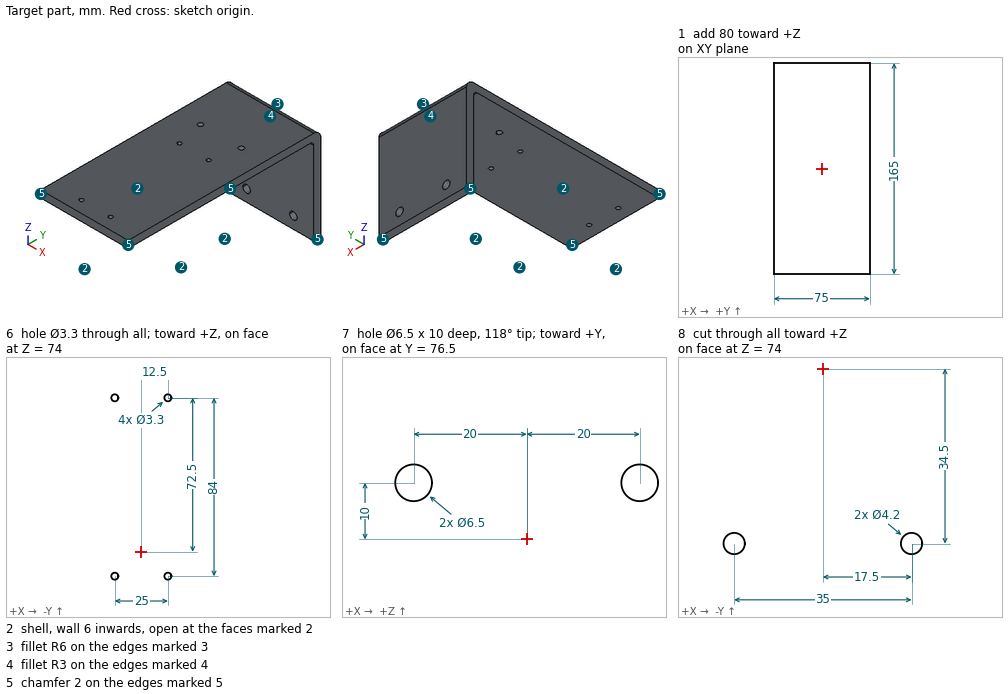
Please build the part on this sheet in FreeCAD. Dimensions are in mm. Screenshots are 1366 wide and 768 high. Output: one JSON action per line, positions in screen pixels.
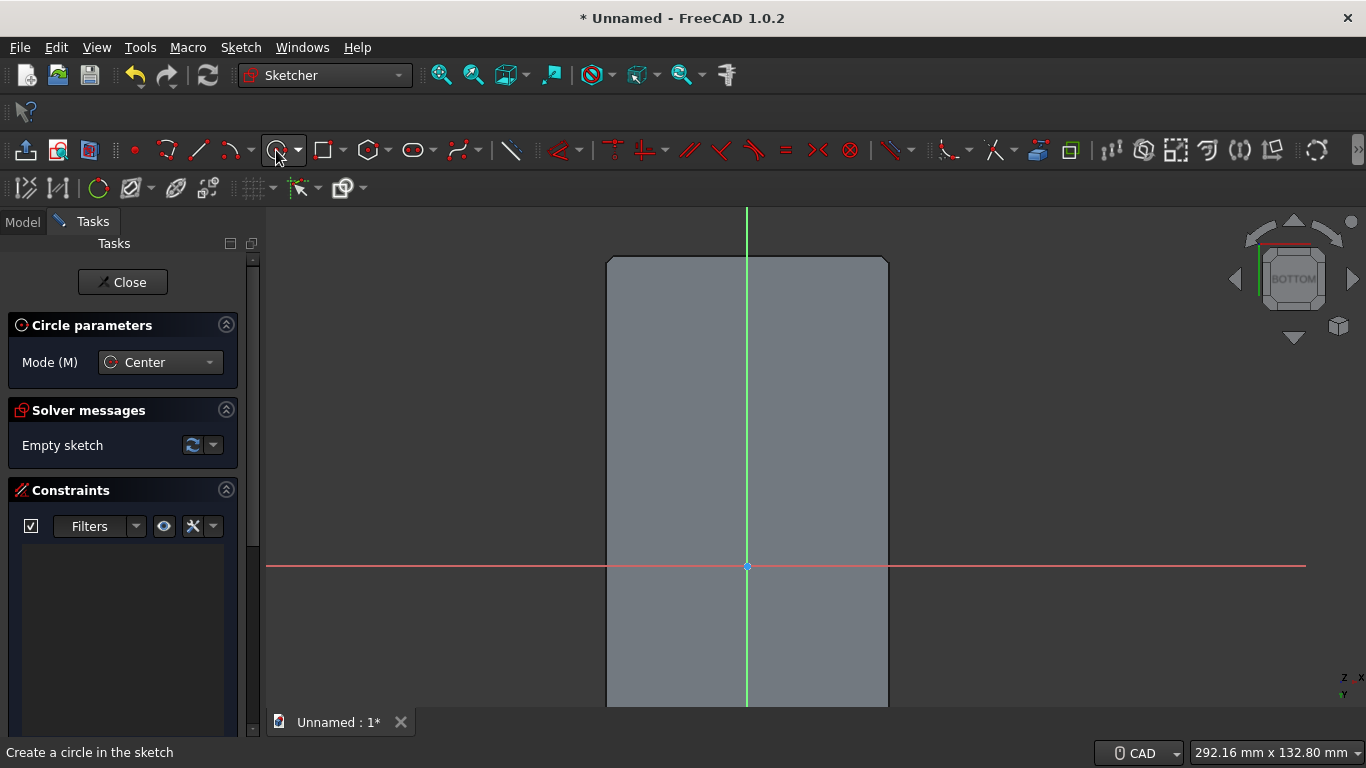
{"action": "scroll", "coordinate": [794, 293], "scroll_direction": "up", "scroll_amount": 7}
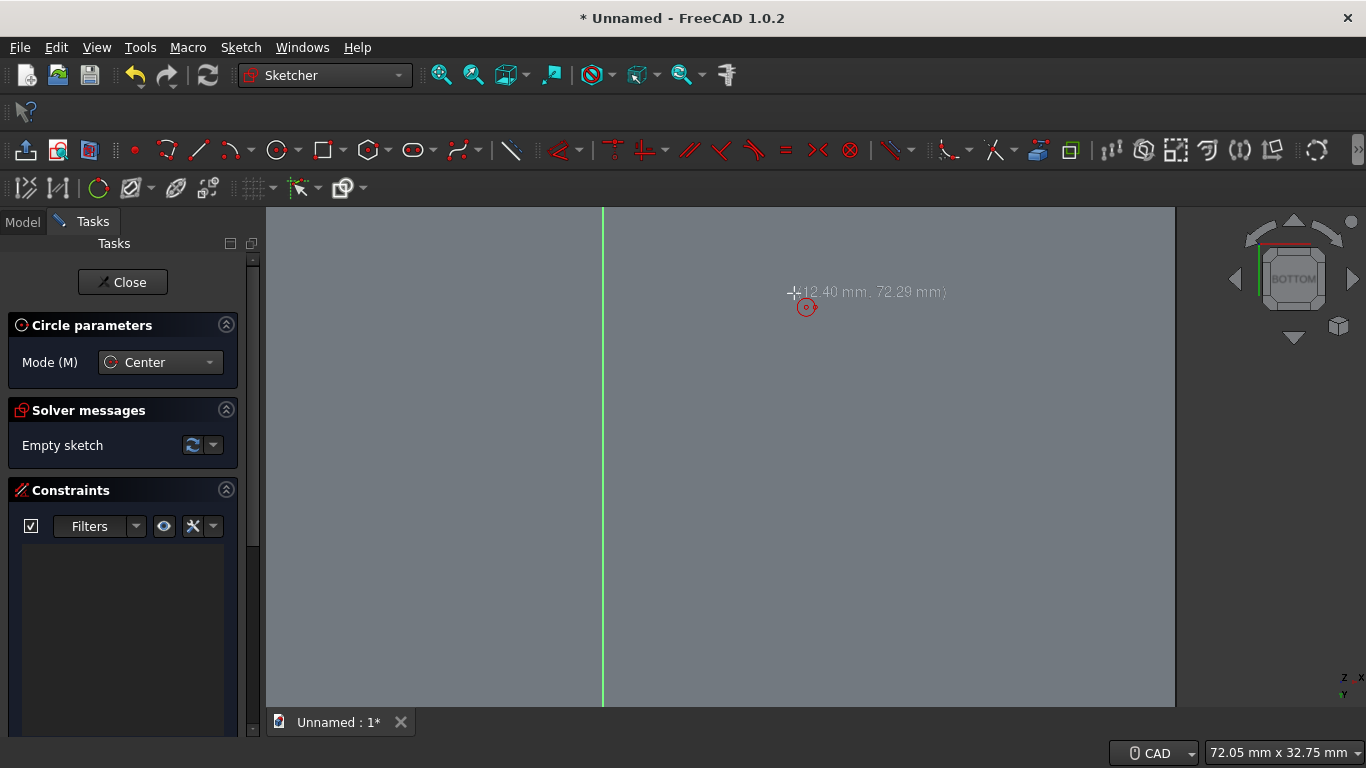
{"action": "scroll", "coordinate": [795, 301], "scroll_direction": "down", "scroll_amount": 7}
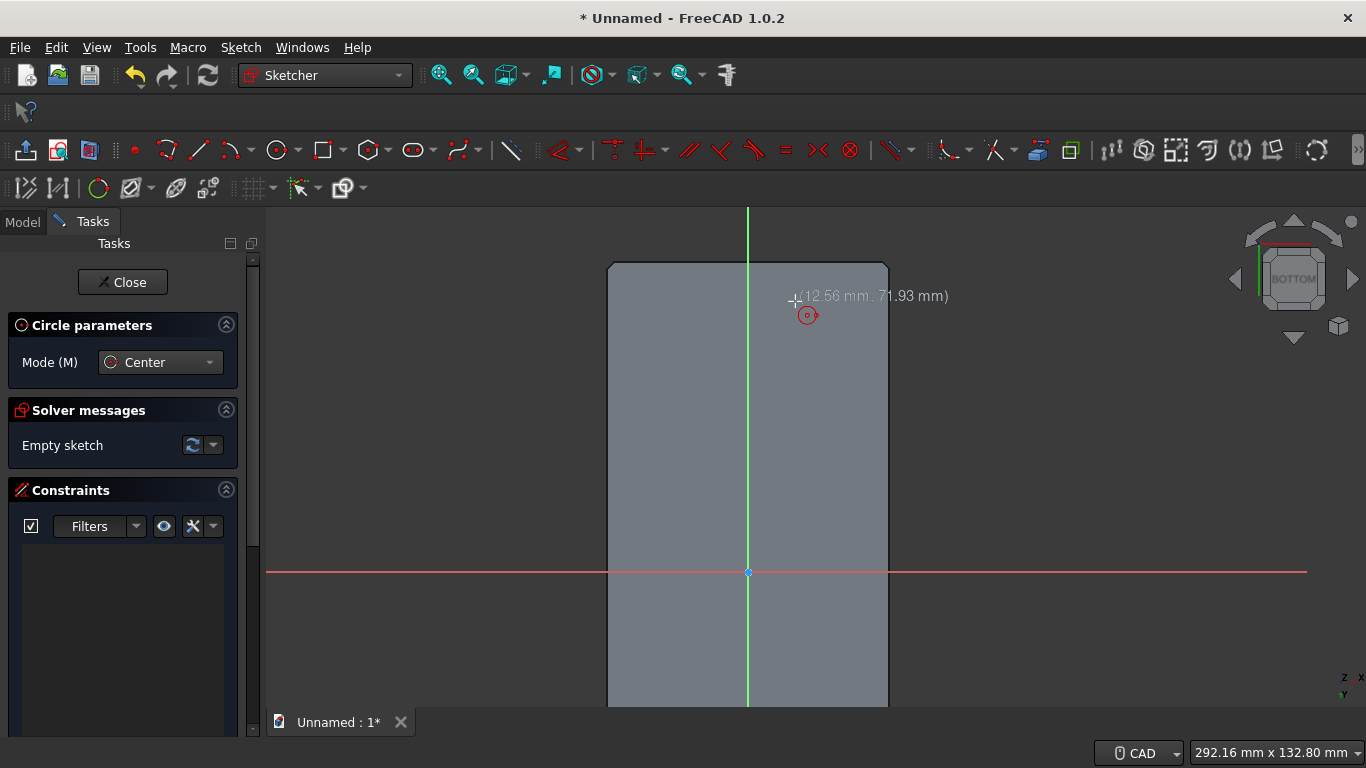
{"action": "left_click", "coordinate": [795, 299]}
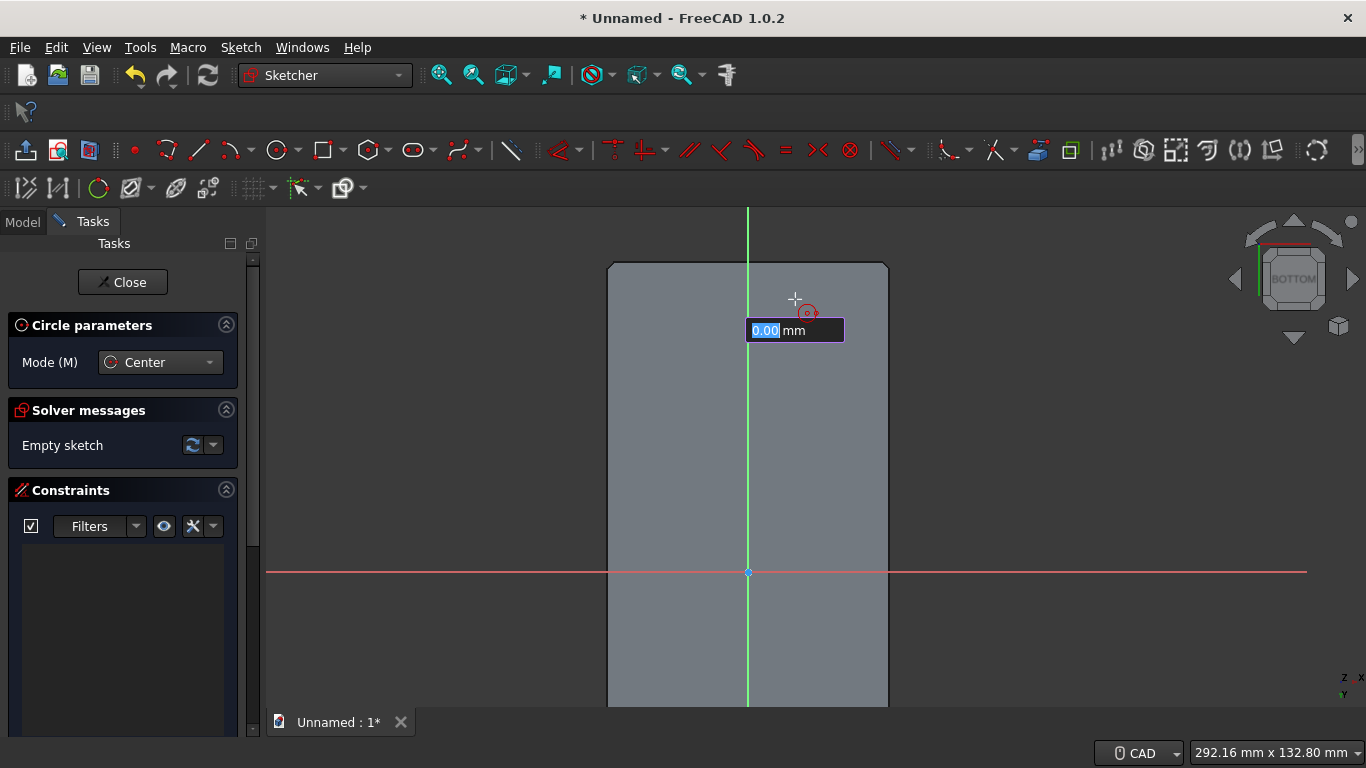
{"action": "scroll", "coordinate": [800, 295], "scroll_direction": "up", "scroll_amount": 5}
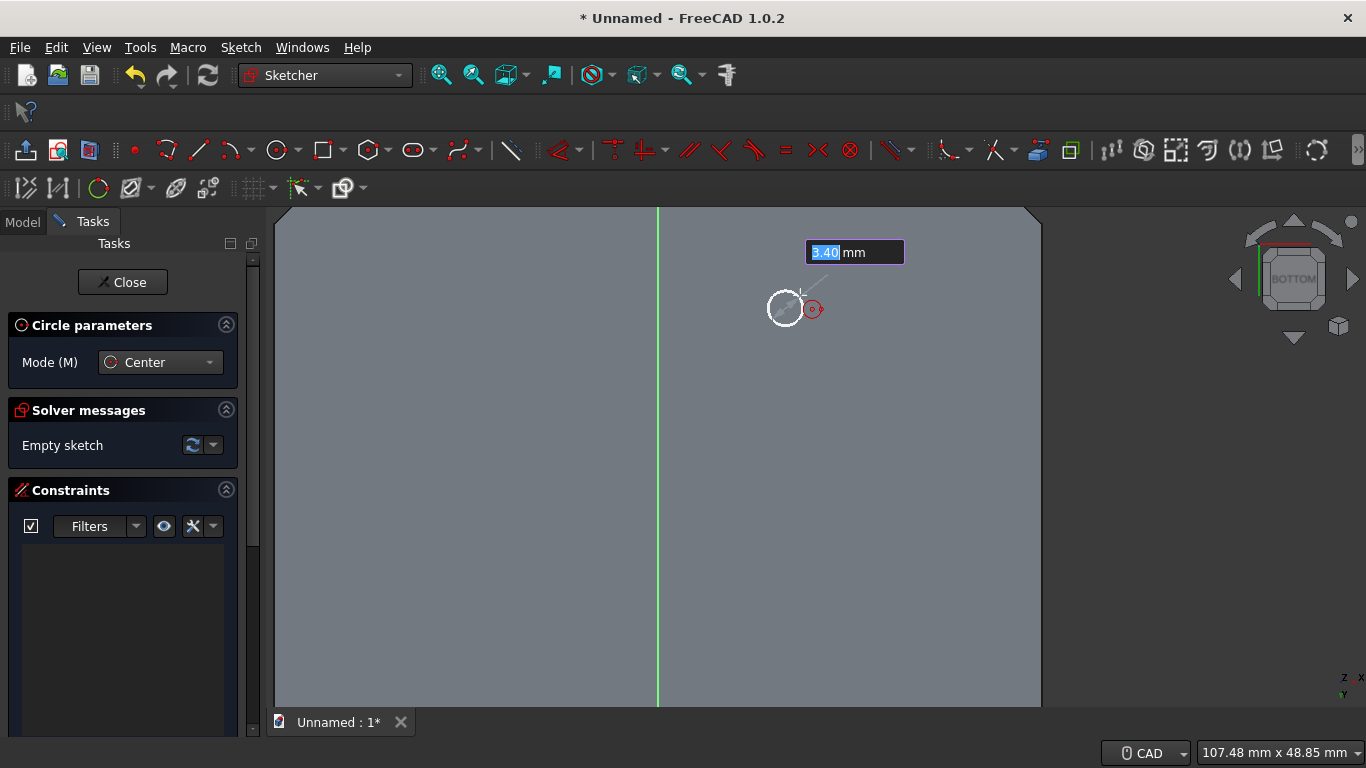
{"action": "left_click", "coordinate": [798, 294]}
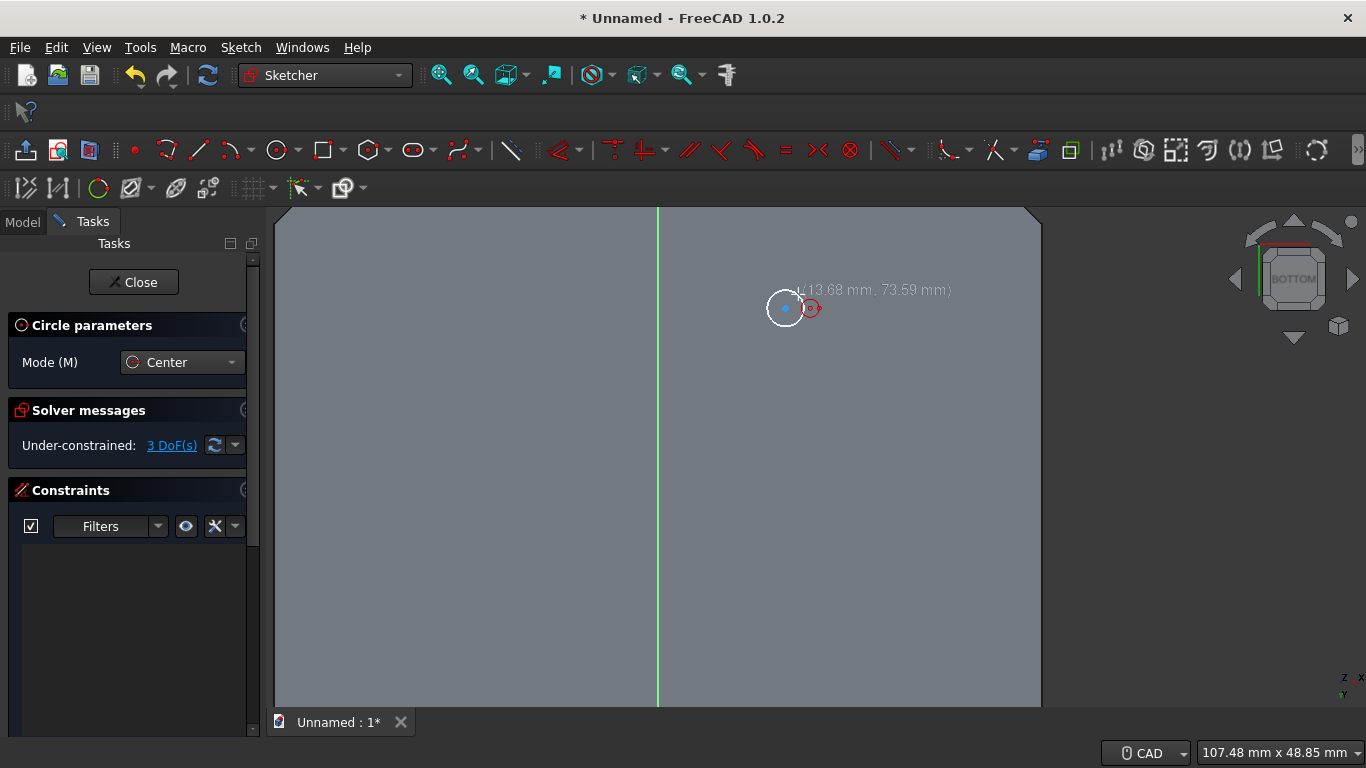
{"action": "scroll", "coordinate": [800, 295], "scroll_direction": "down", "scroll_amount": 5}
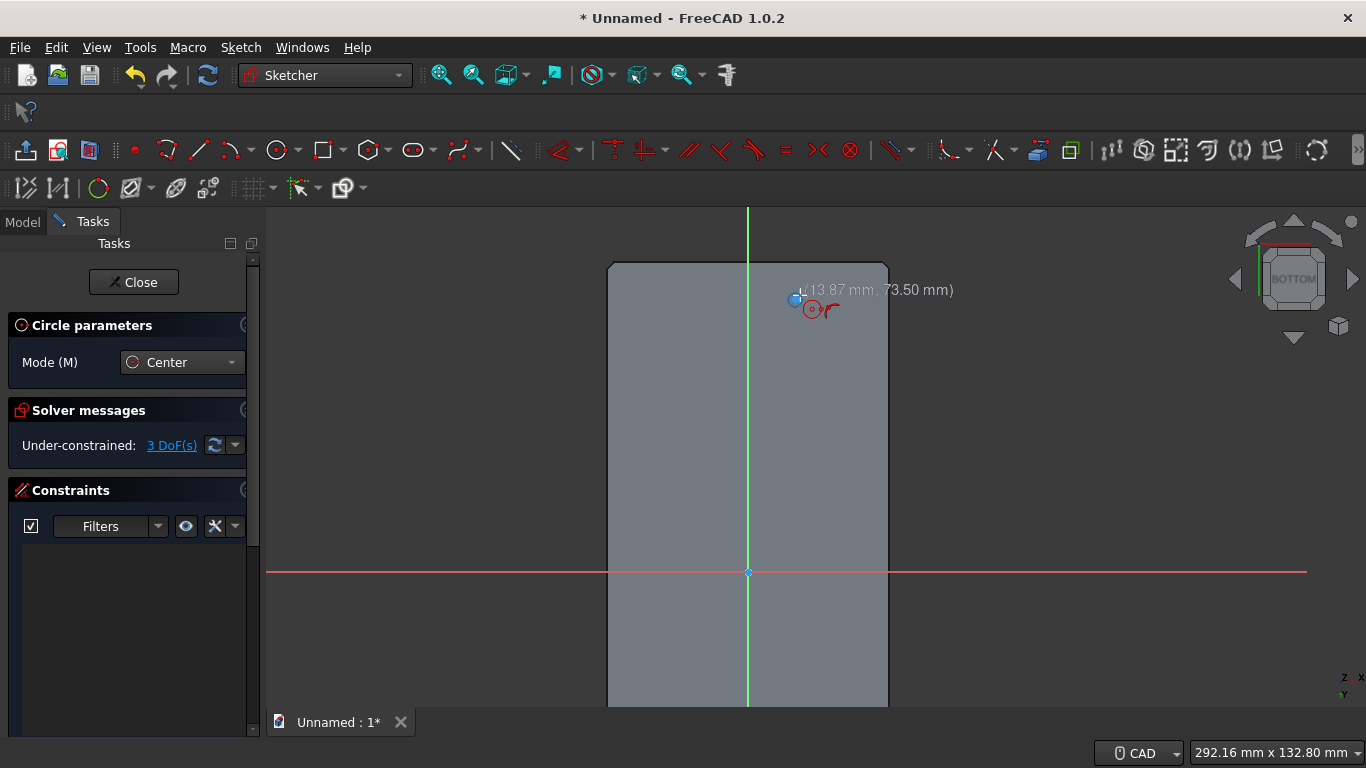
{"action": "scroll", "coordinate": [795, 615], "scroll_direction": "up", "scroll_amount": 7}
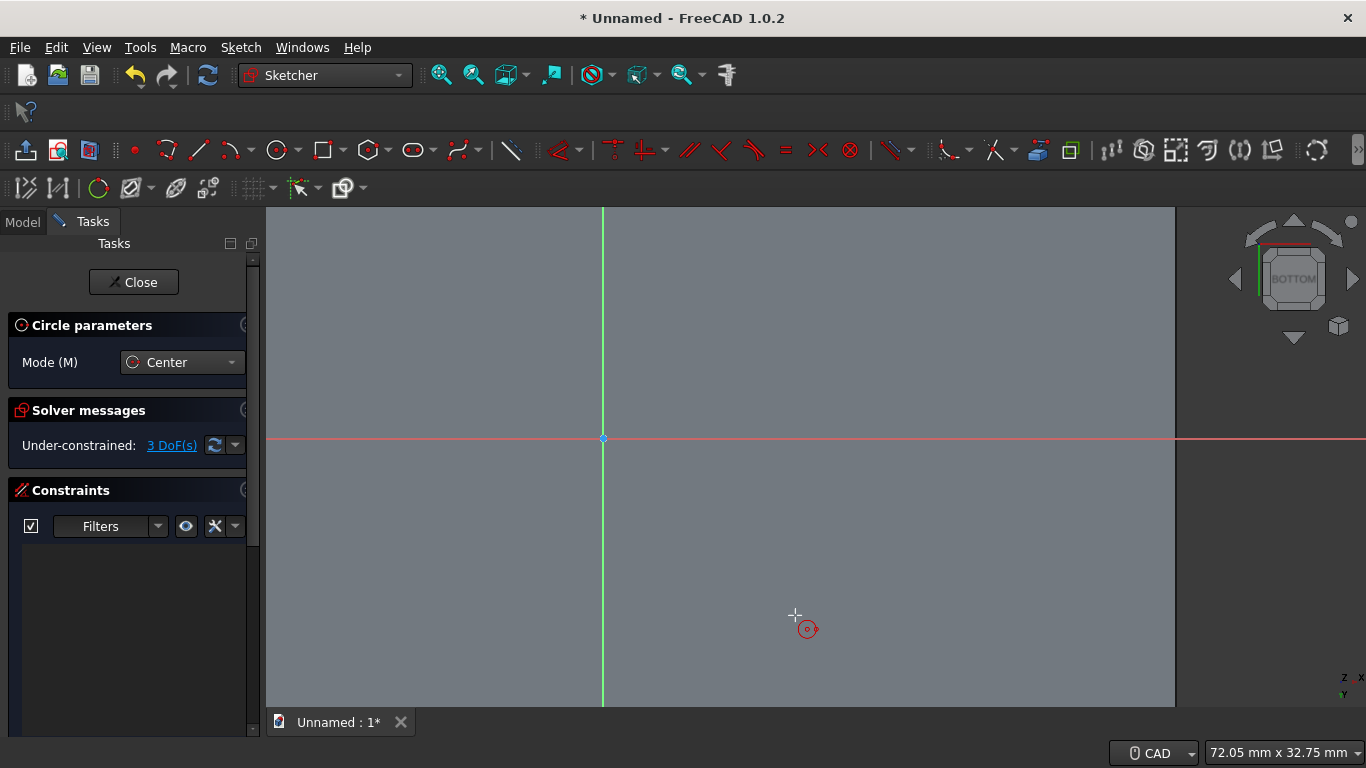
{"action": "scroll", "coordinate": [795, 615], "scroll_direction": "down", "scroll_amount": 7}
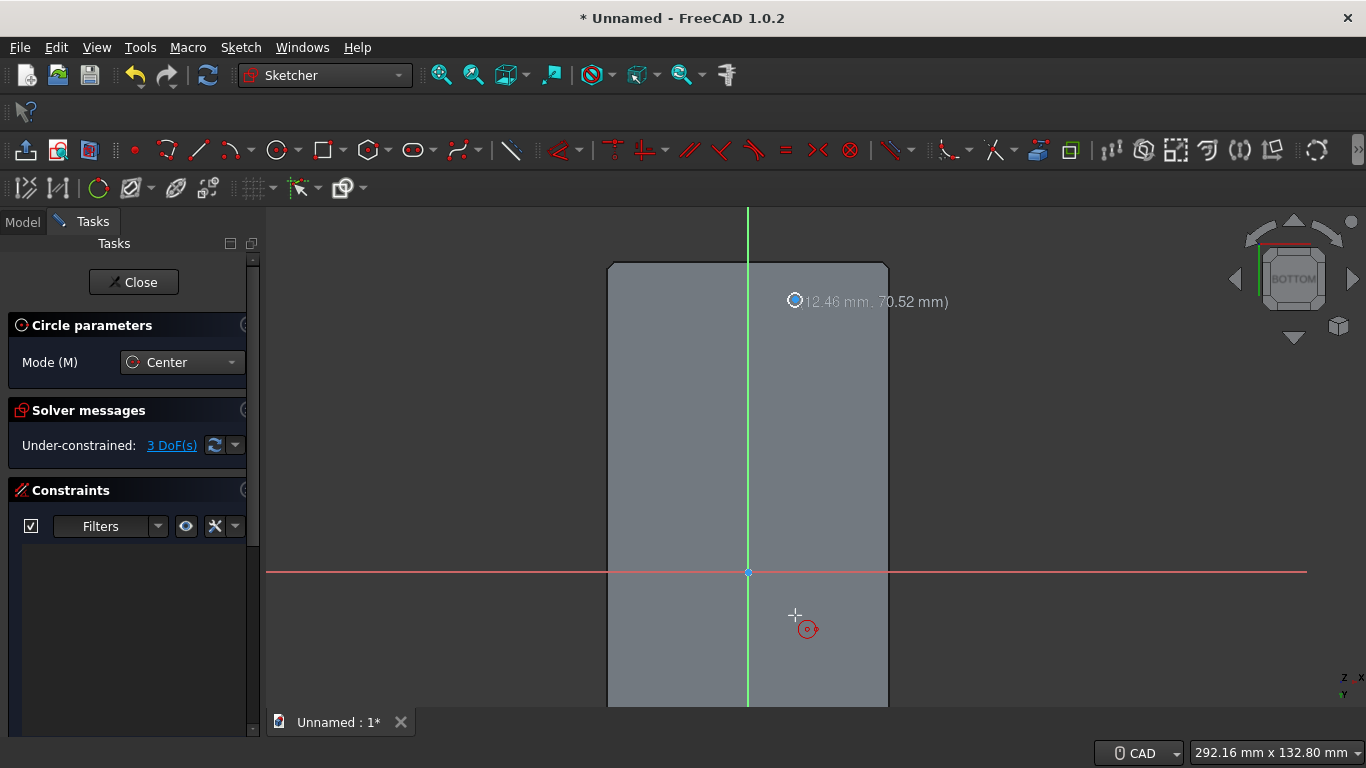
{"action": "left_click", "coordinate": [795, 615]}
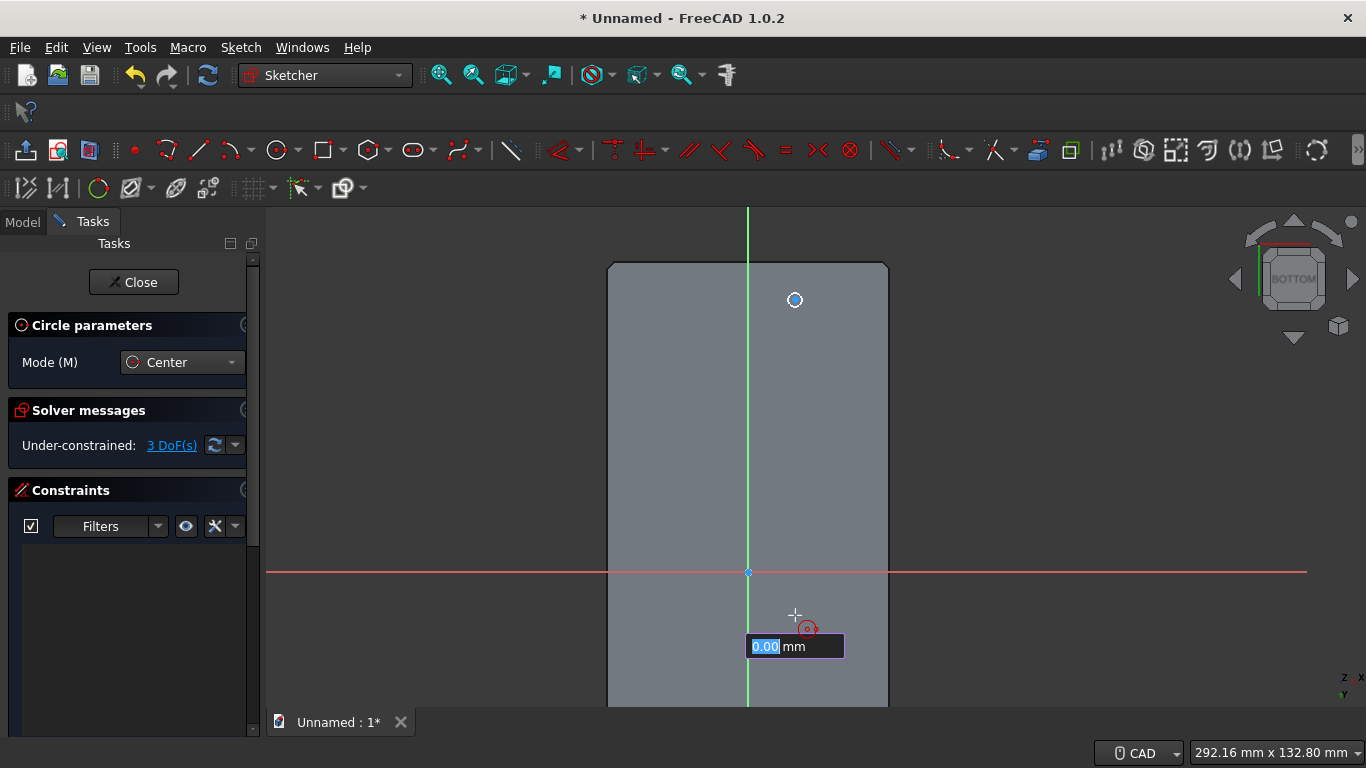
{"action": "scroll", "coordinate": [800, 611], "scroll_direction": "up", "scroll_amount": 5}